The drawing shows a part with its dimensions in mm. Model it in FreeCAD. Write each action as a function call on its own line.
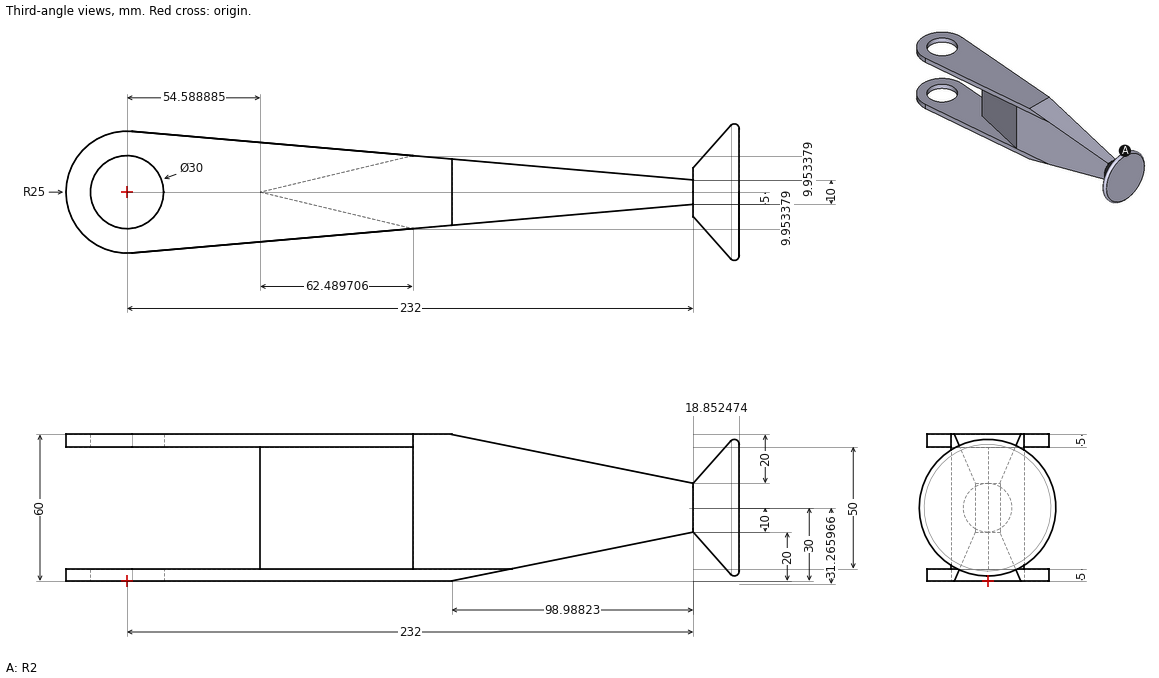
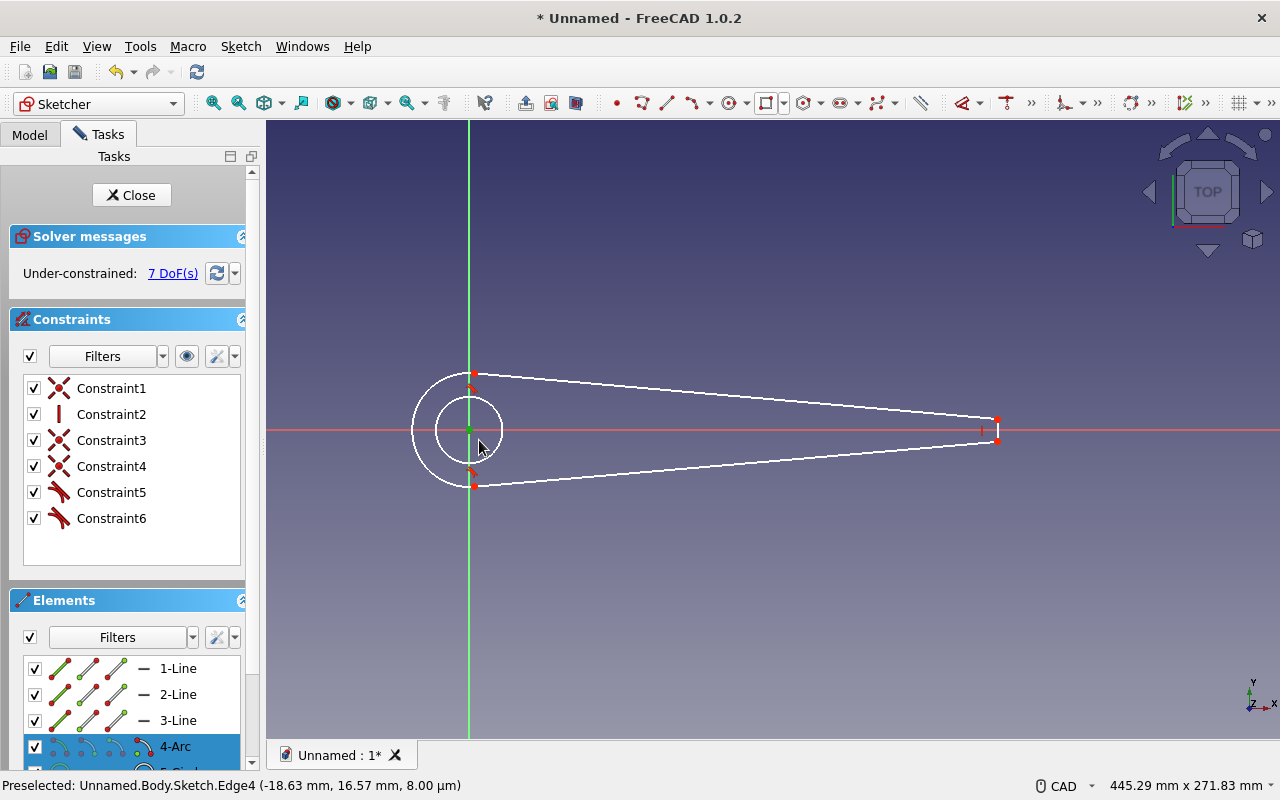
click(1006, 104)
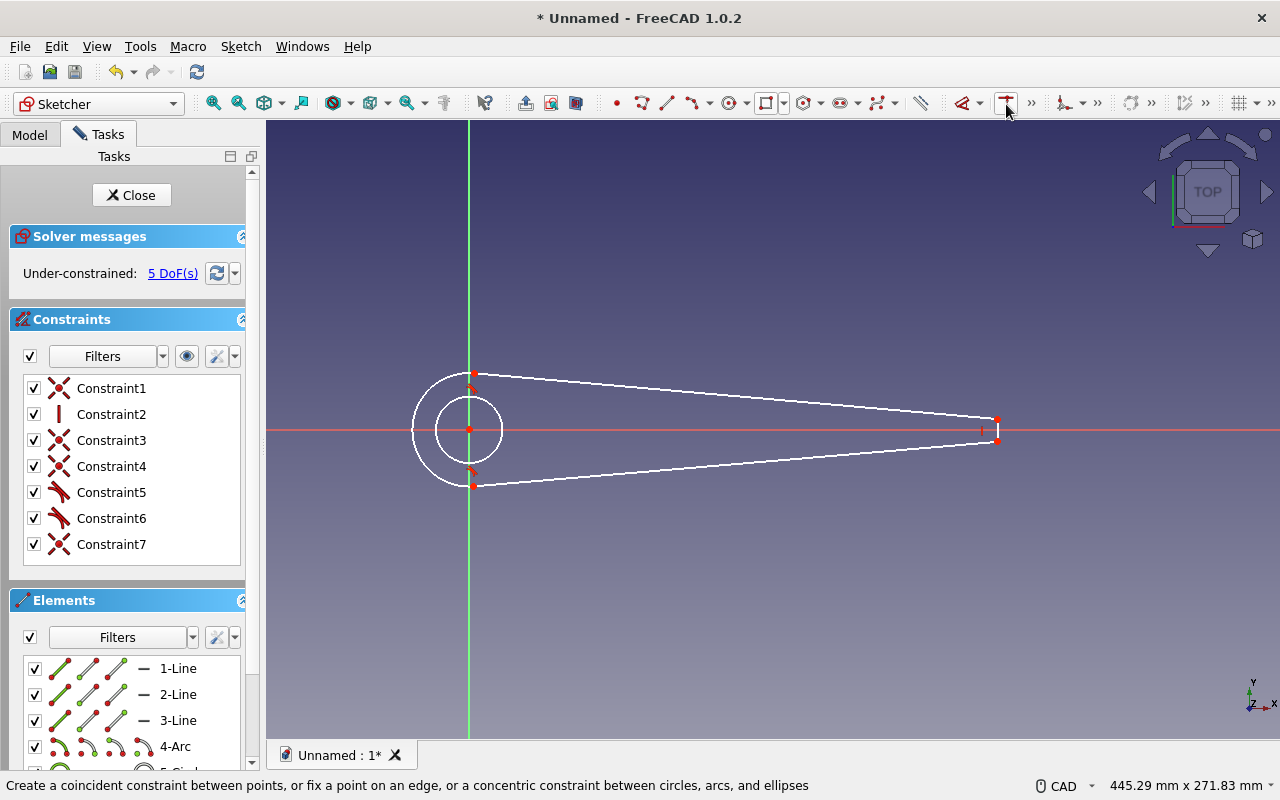
click(962, 104)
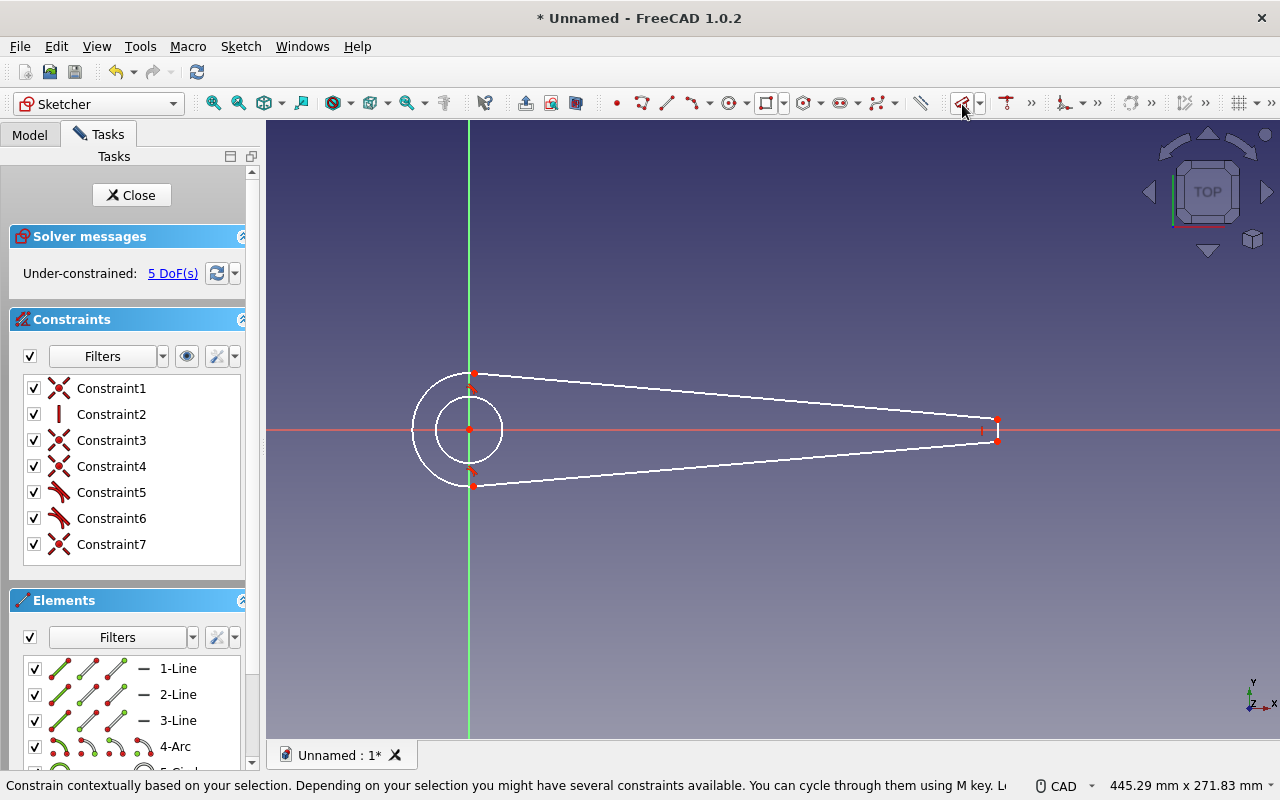
click(424, 395)
click(399, 375)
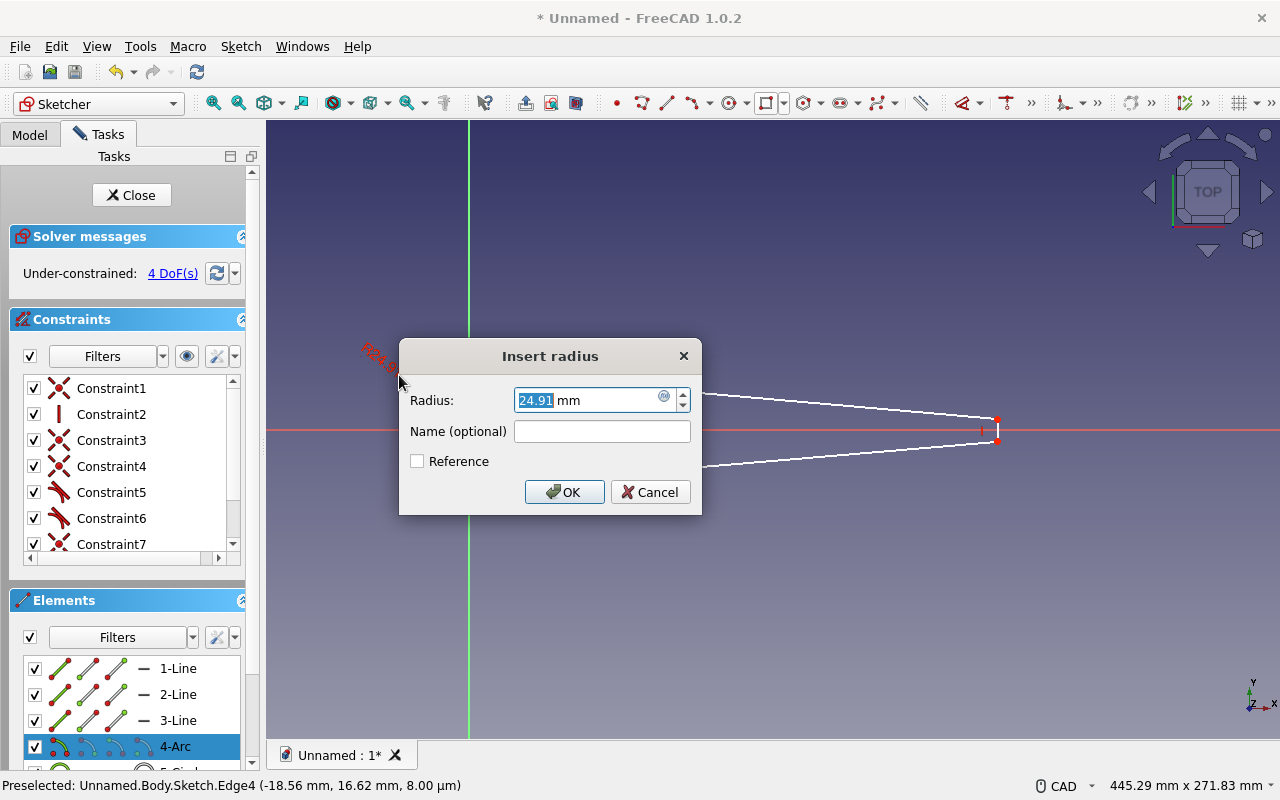
text(25)
key(Return)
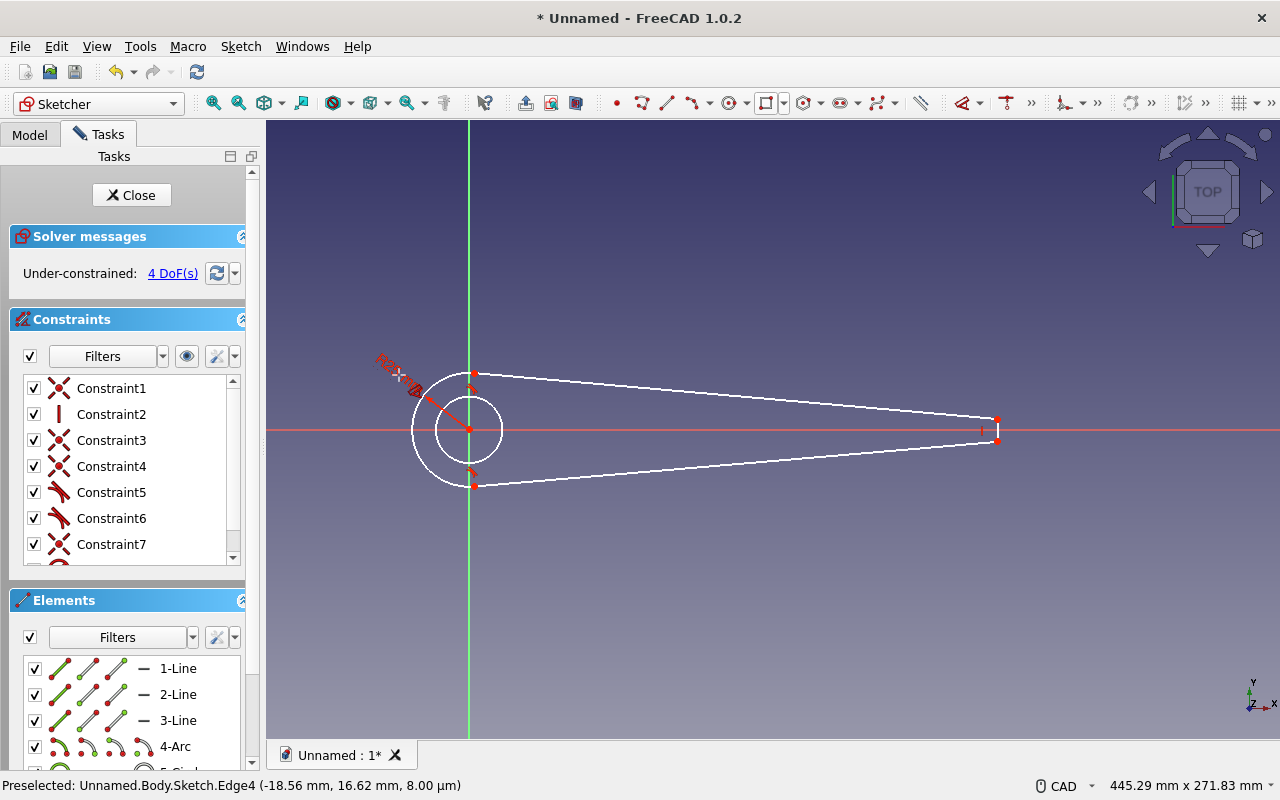
click(493, 406)
click(532, 411)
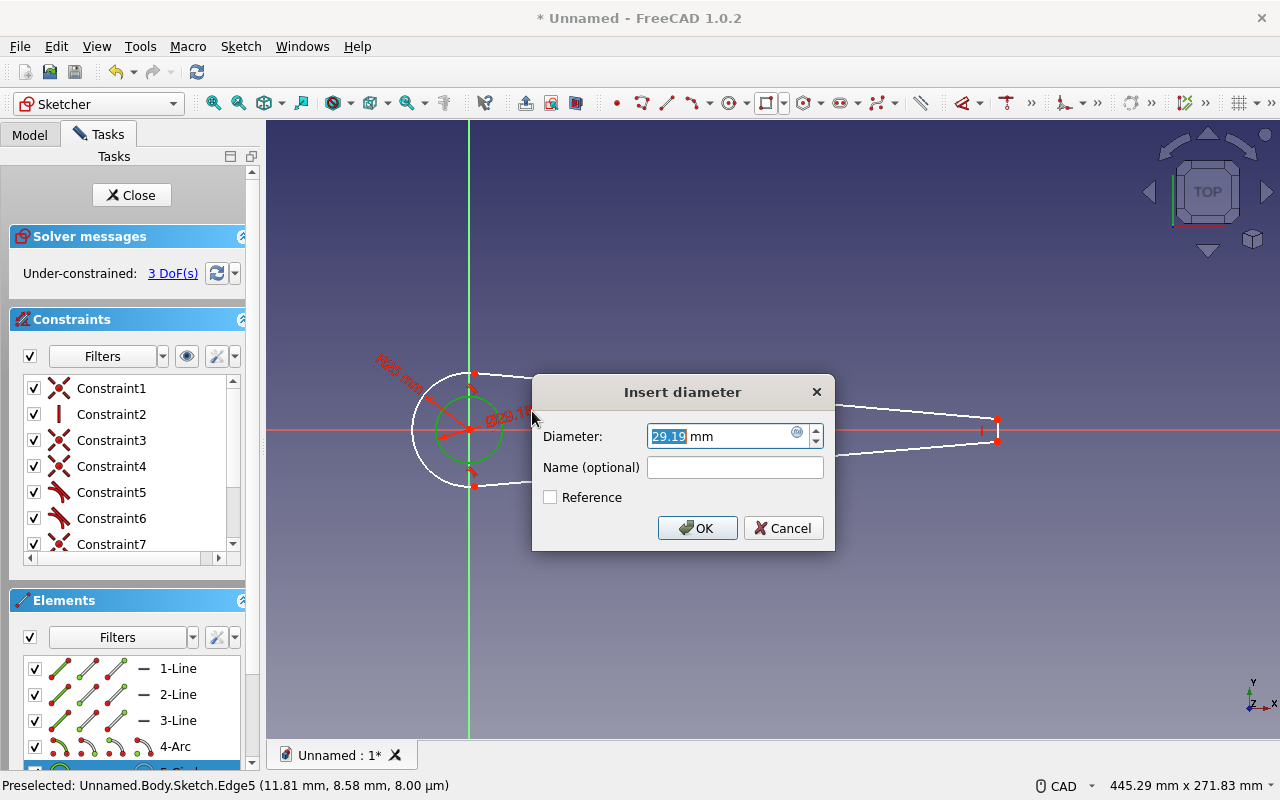
text(30)
key(Return)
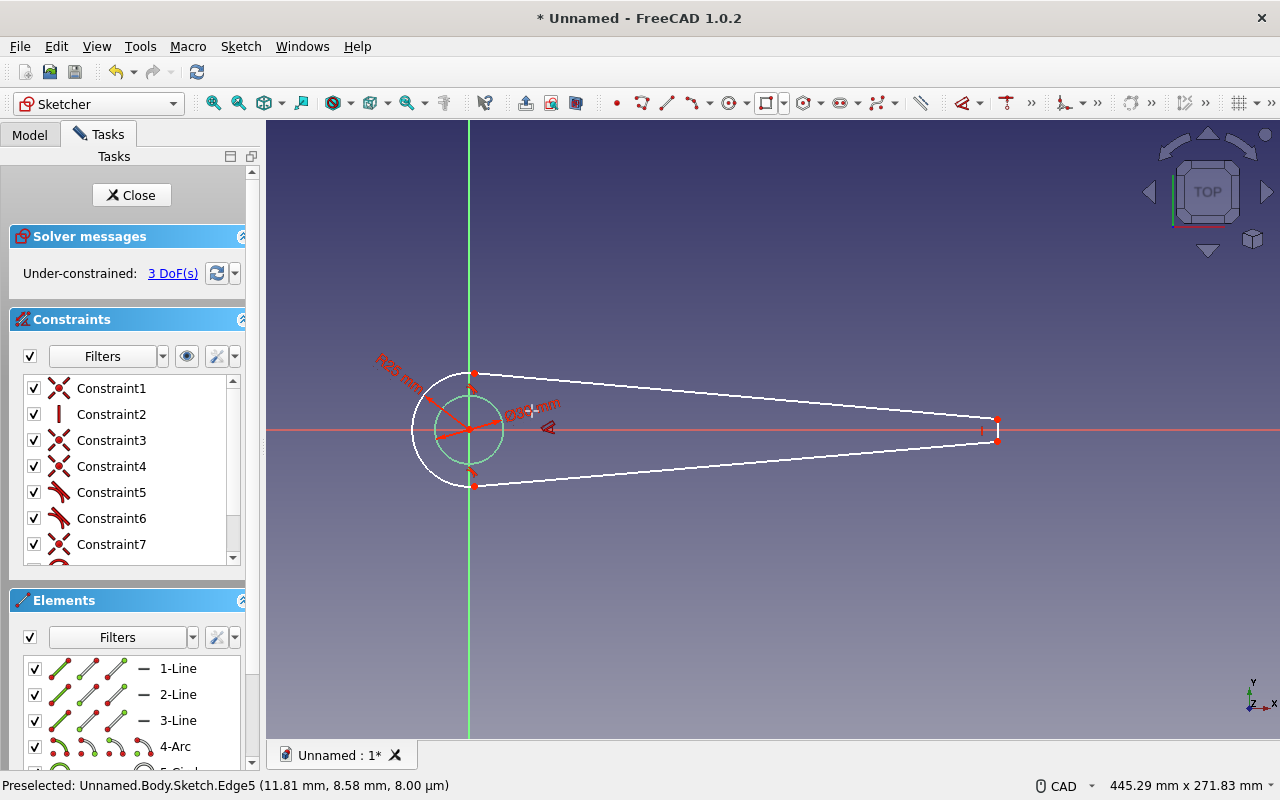
scroll(998, 433, up, 3)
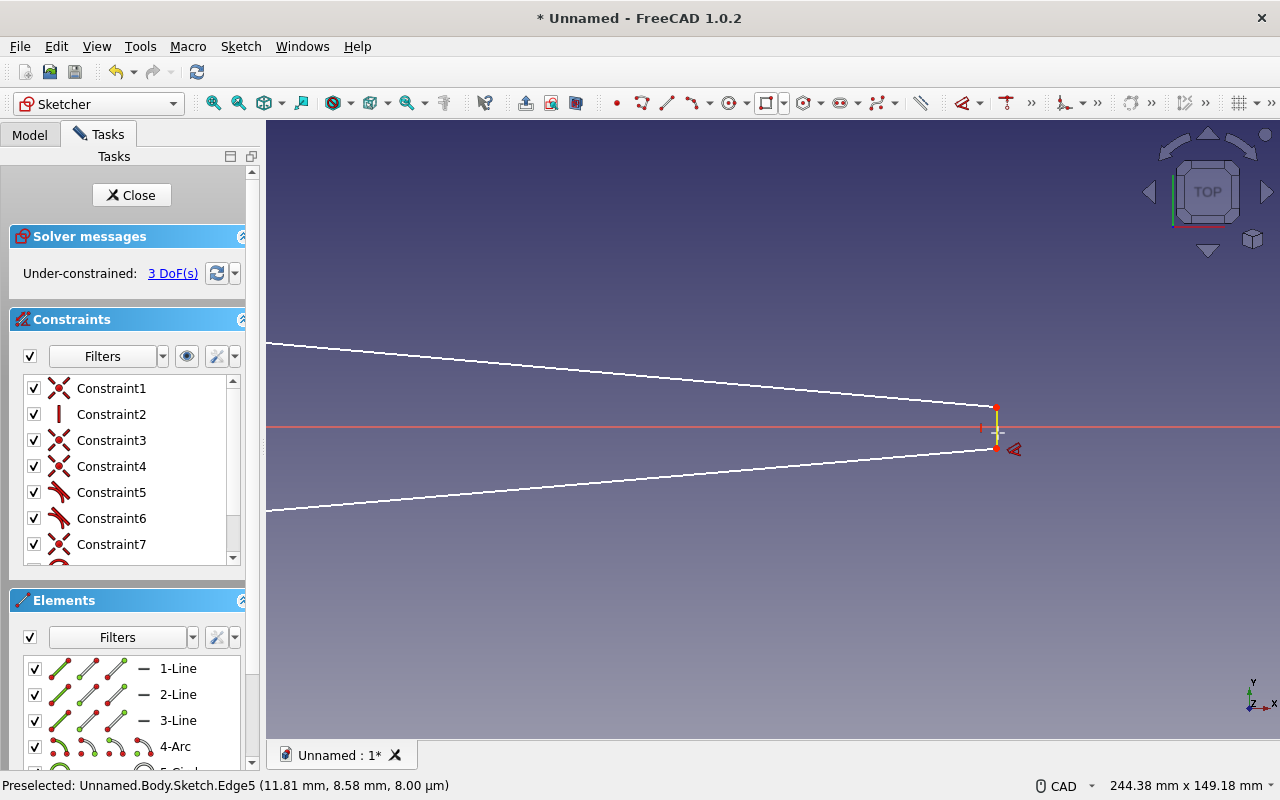
click(997, 432)
click(1031, 413)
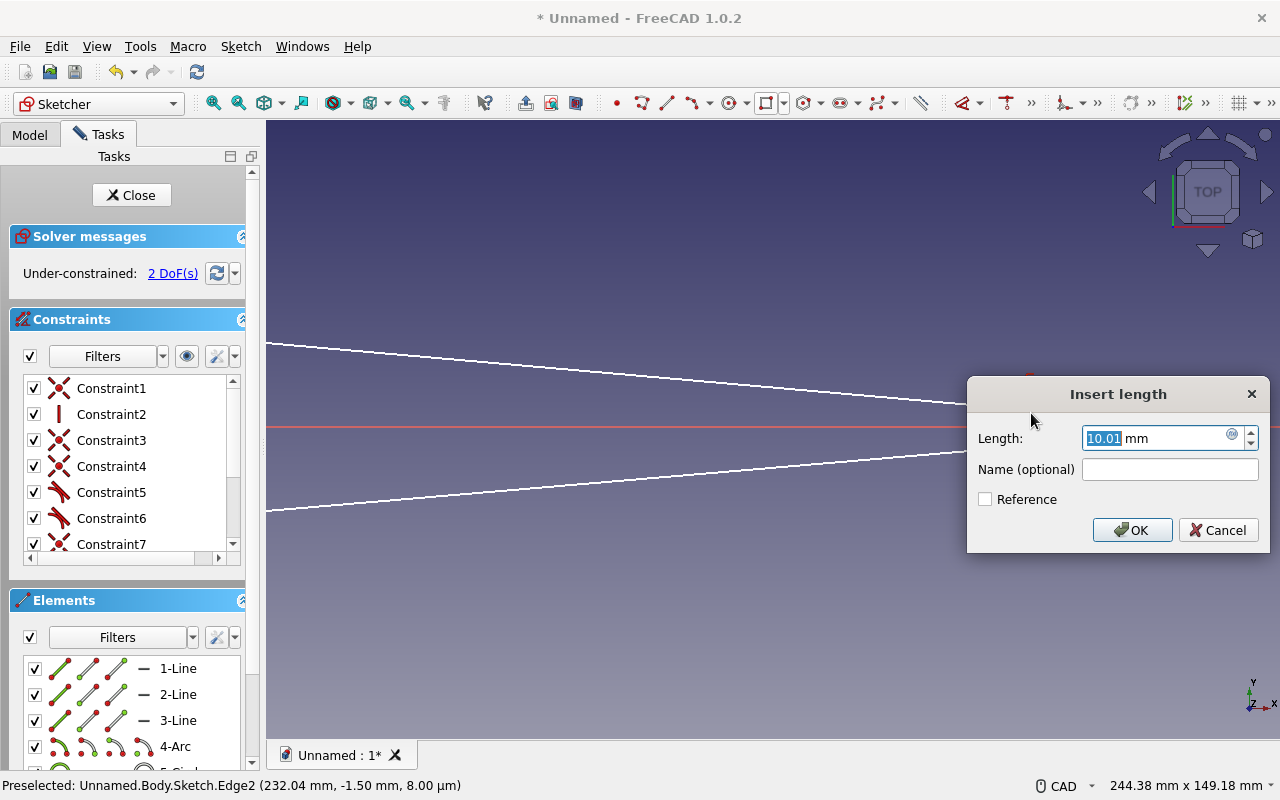
text(10)
key(Return)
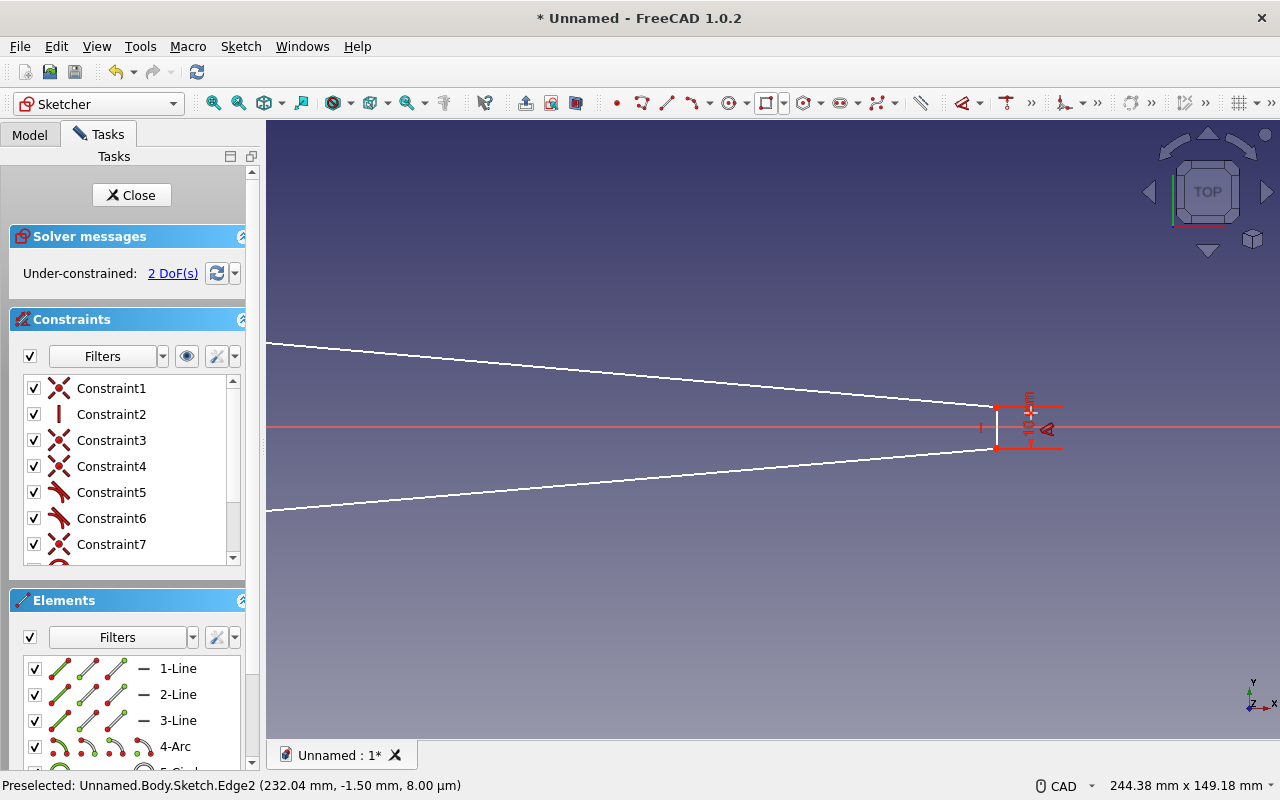
scroll(997, 449, up, 4)